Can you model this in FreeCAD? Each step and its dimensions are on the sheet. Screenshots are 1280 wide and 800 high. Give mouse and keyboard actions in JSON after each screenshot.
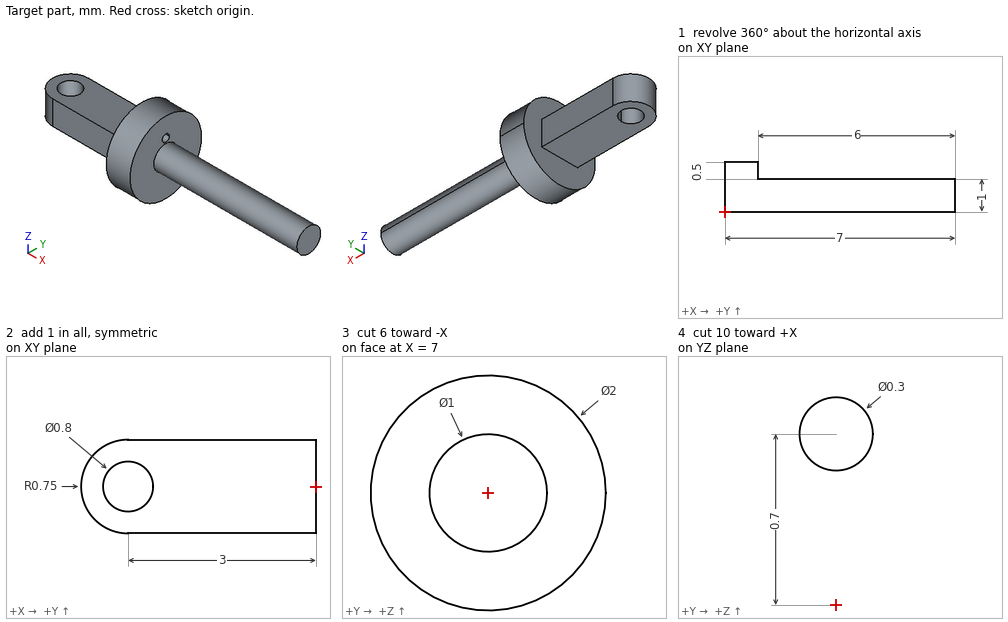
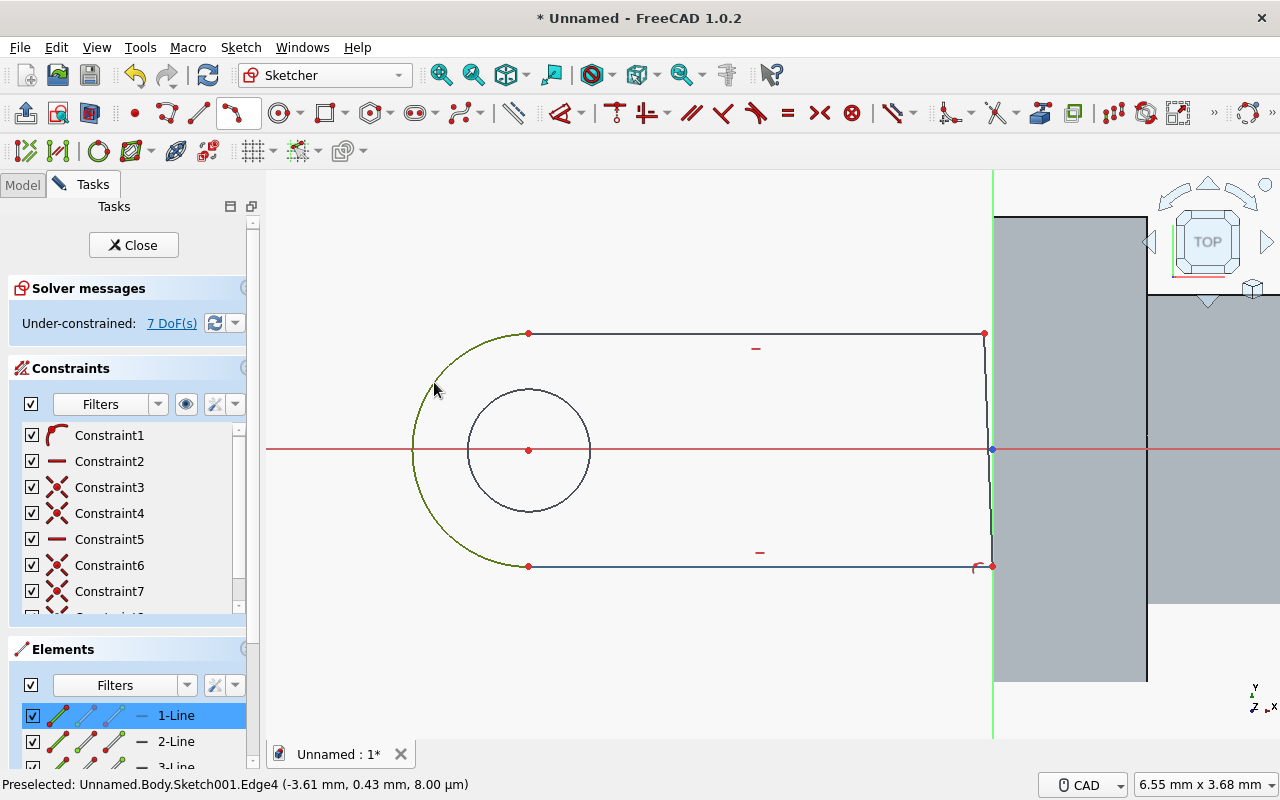
{"action": "left_click", "coordinate": [756, 114]}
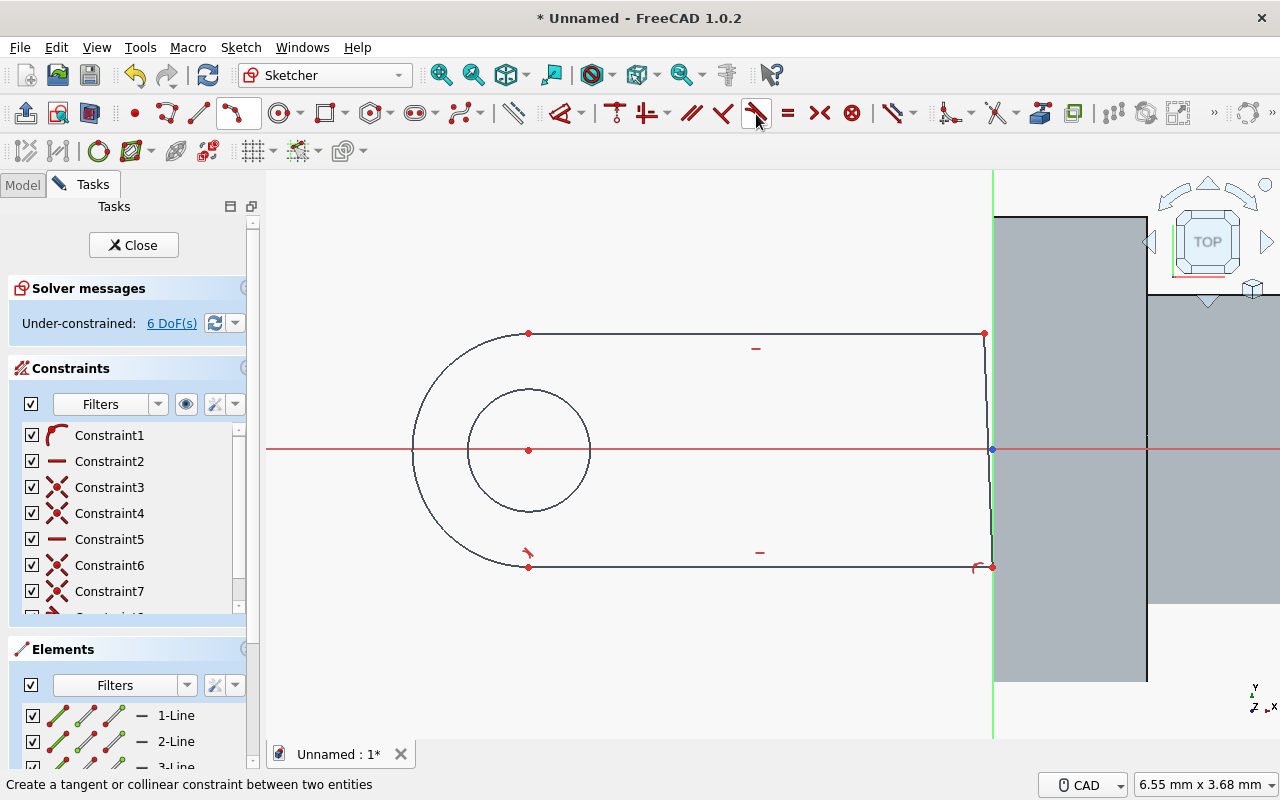
{"action": "left_click", "coordinate": [847, 334]}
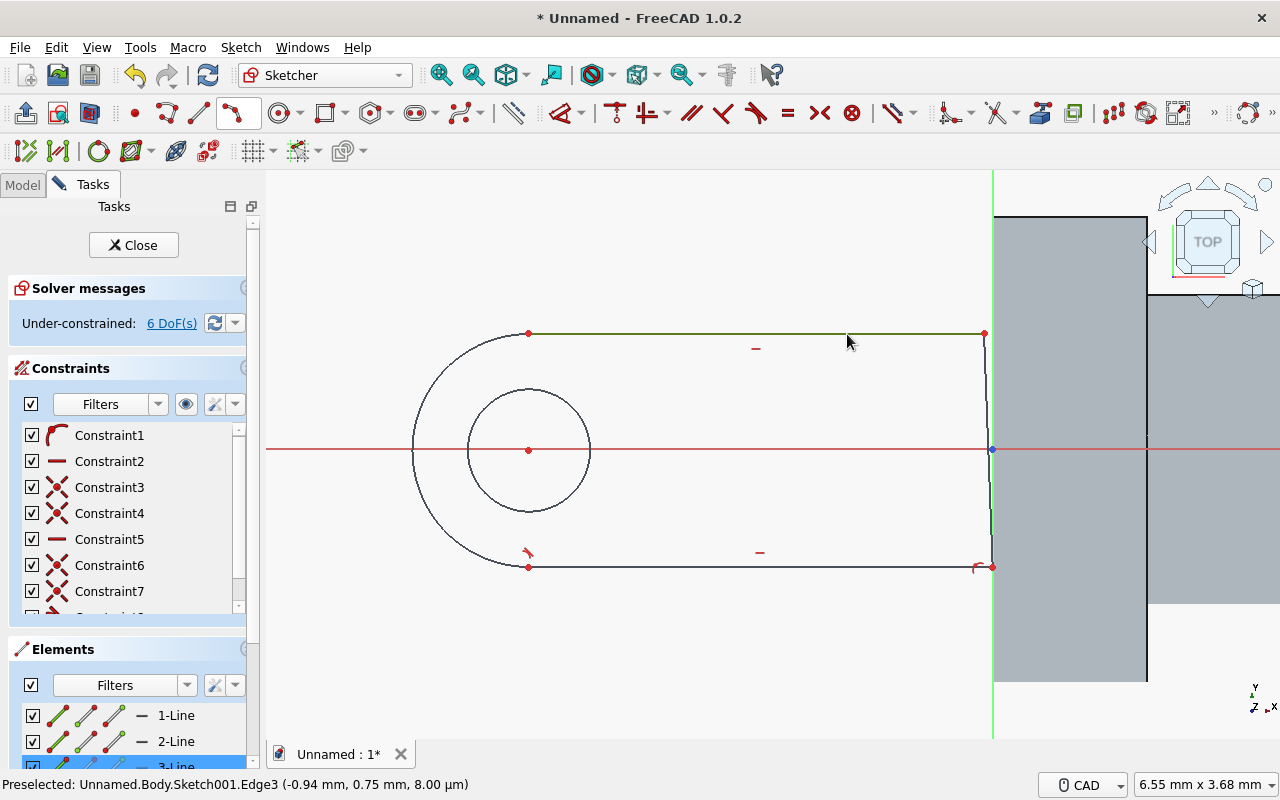
{"action": "left_click", "coordinate": [434, 383]}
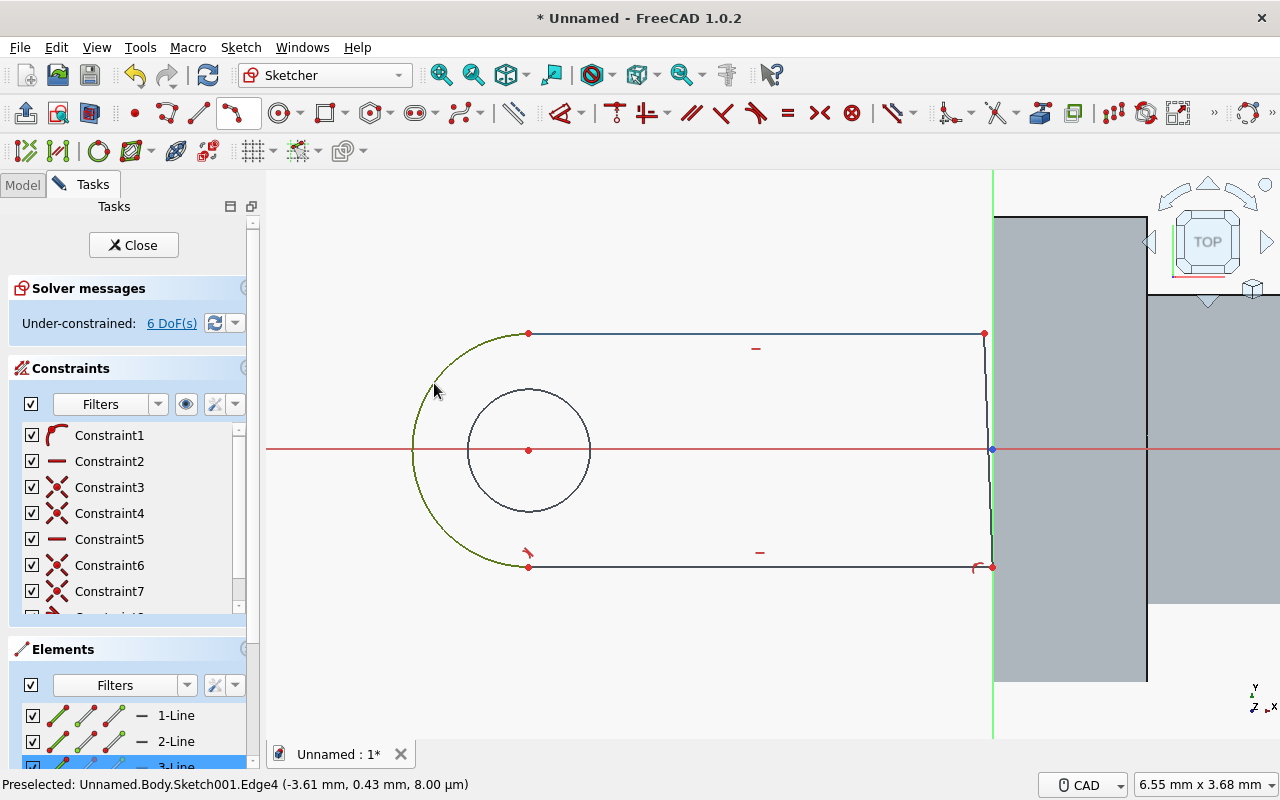
{"action": "left_click", "coordinate": [756, 114]}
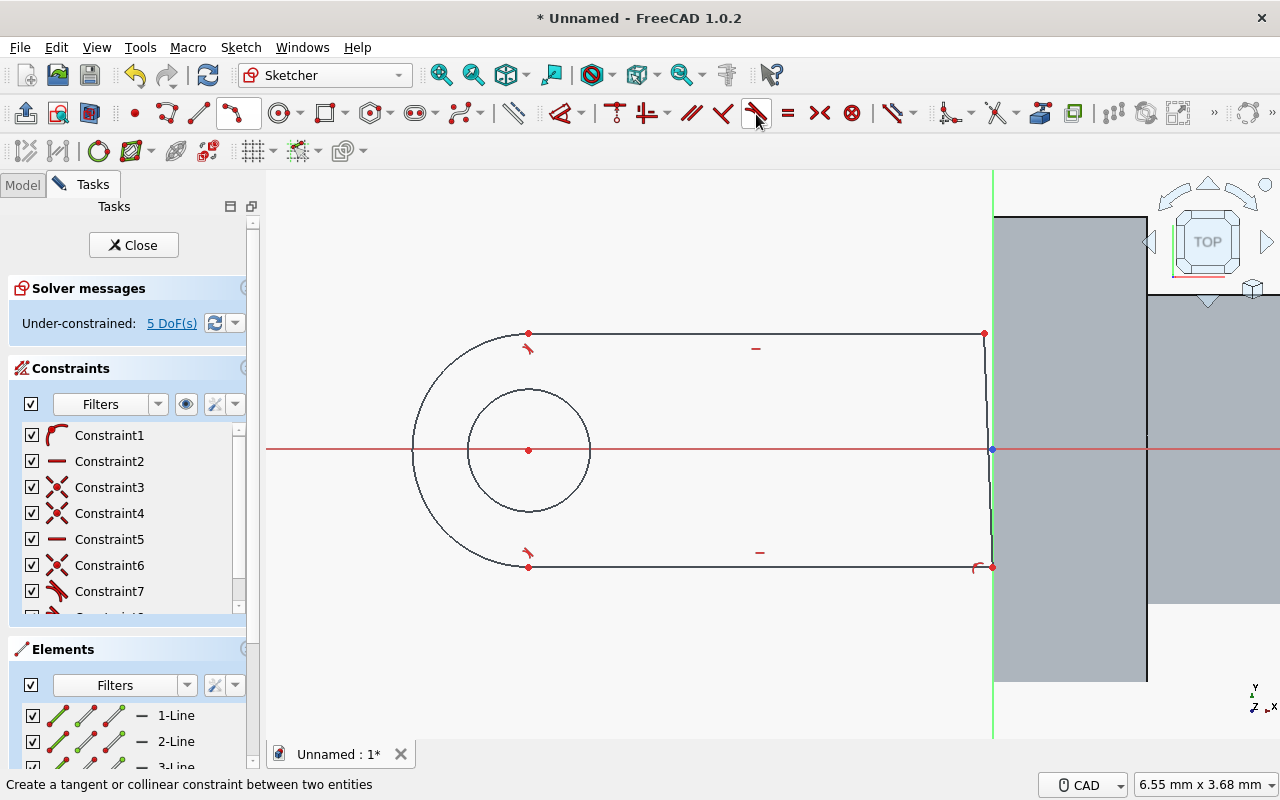
{"action": "left_click", "coordinate": [990, 497]}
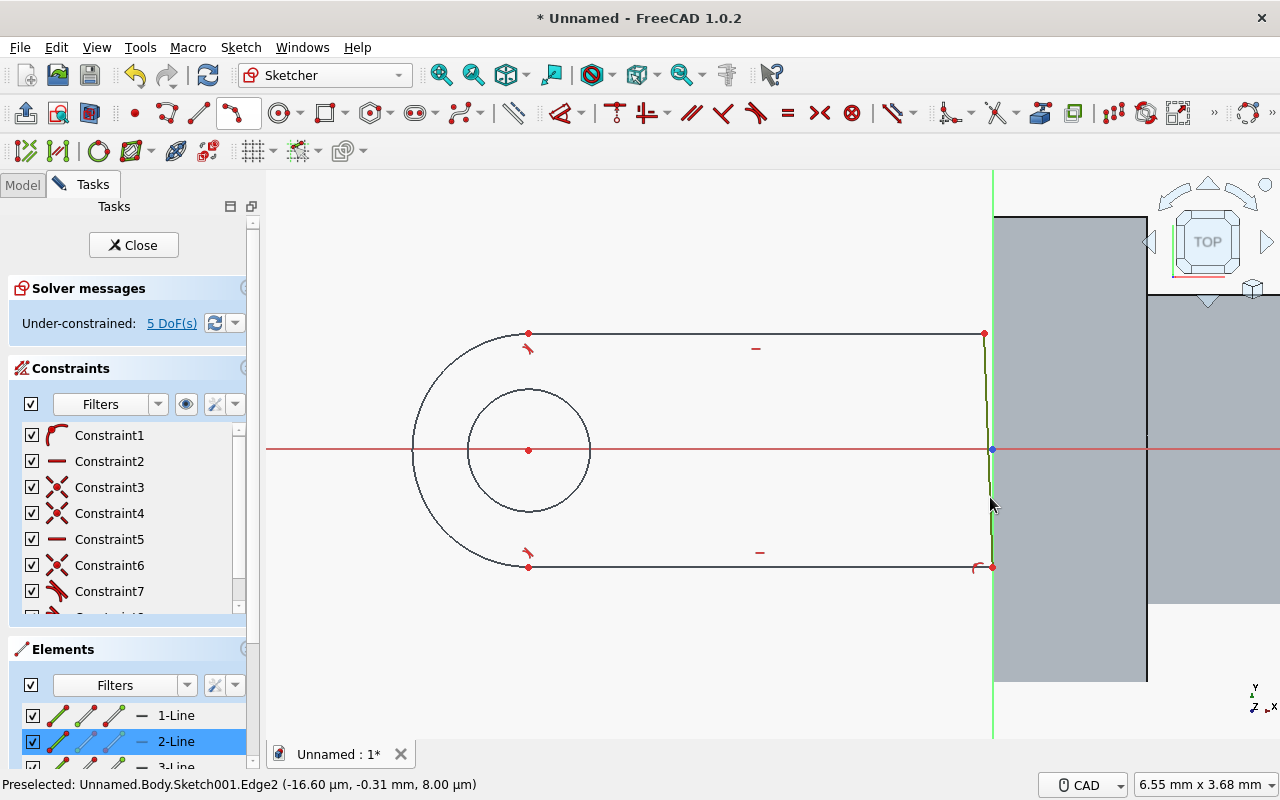
{"action": "left_click", "coordinate": [670, 114]}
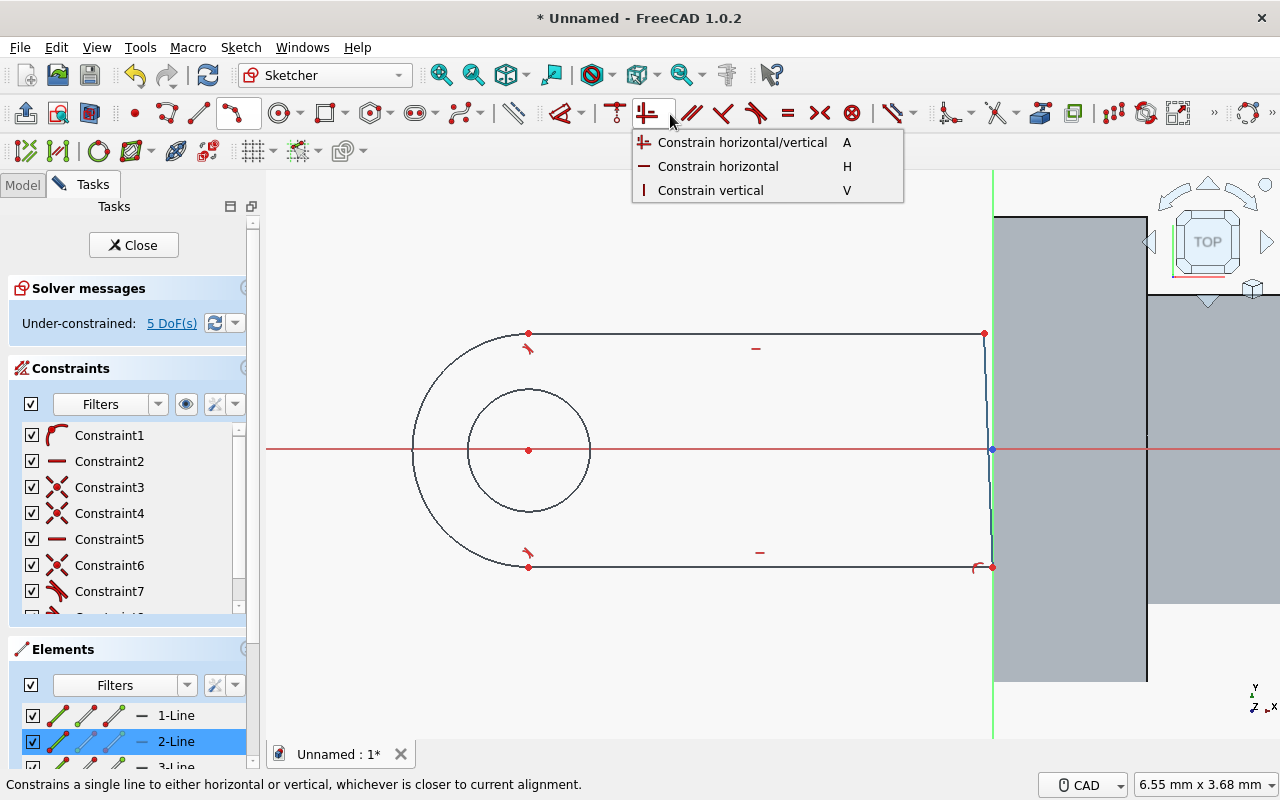
{"action": "left_click", "coordinate": [768, 190]}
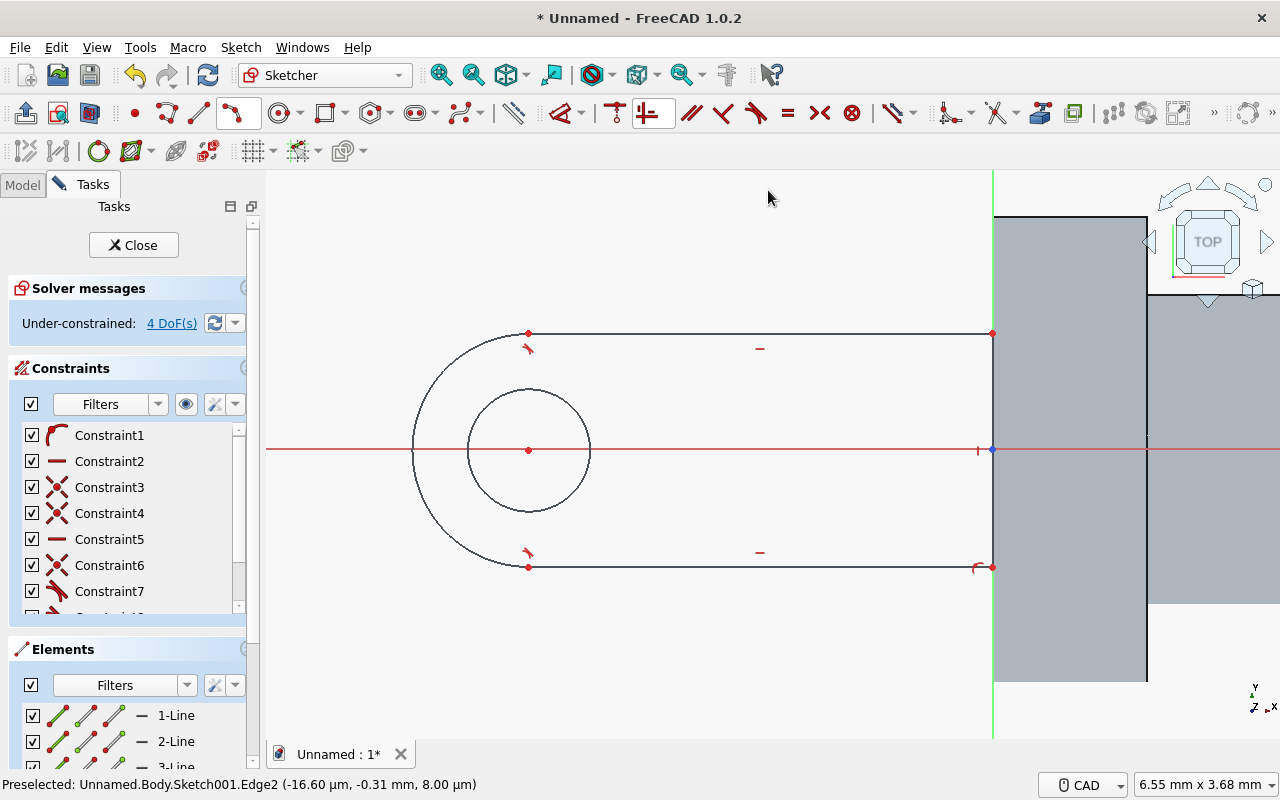
{"action": "left_click", "coordinate": [529, 451]}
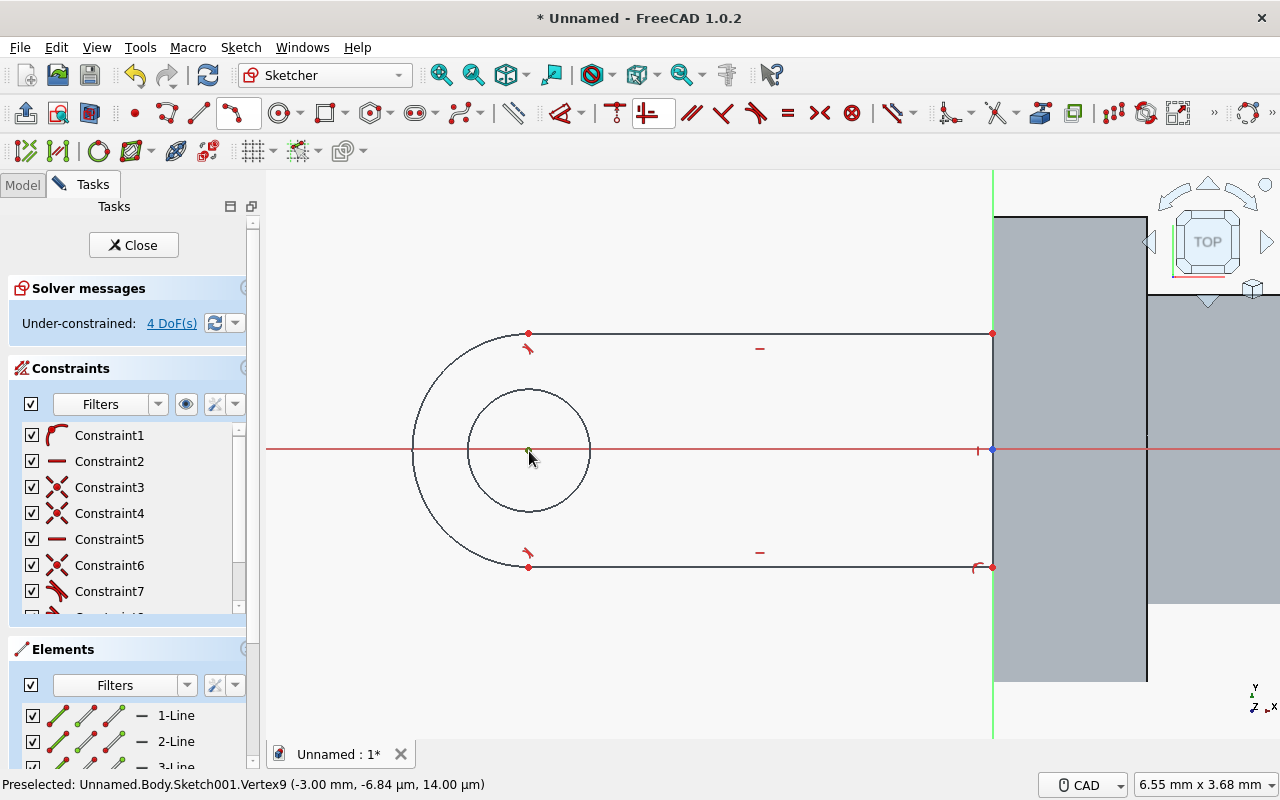
{"action": "left_click", "coordinate": [353, 449]}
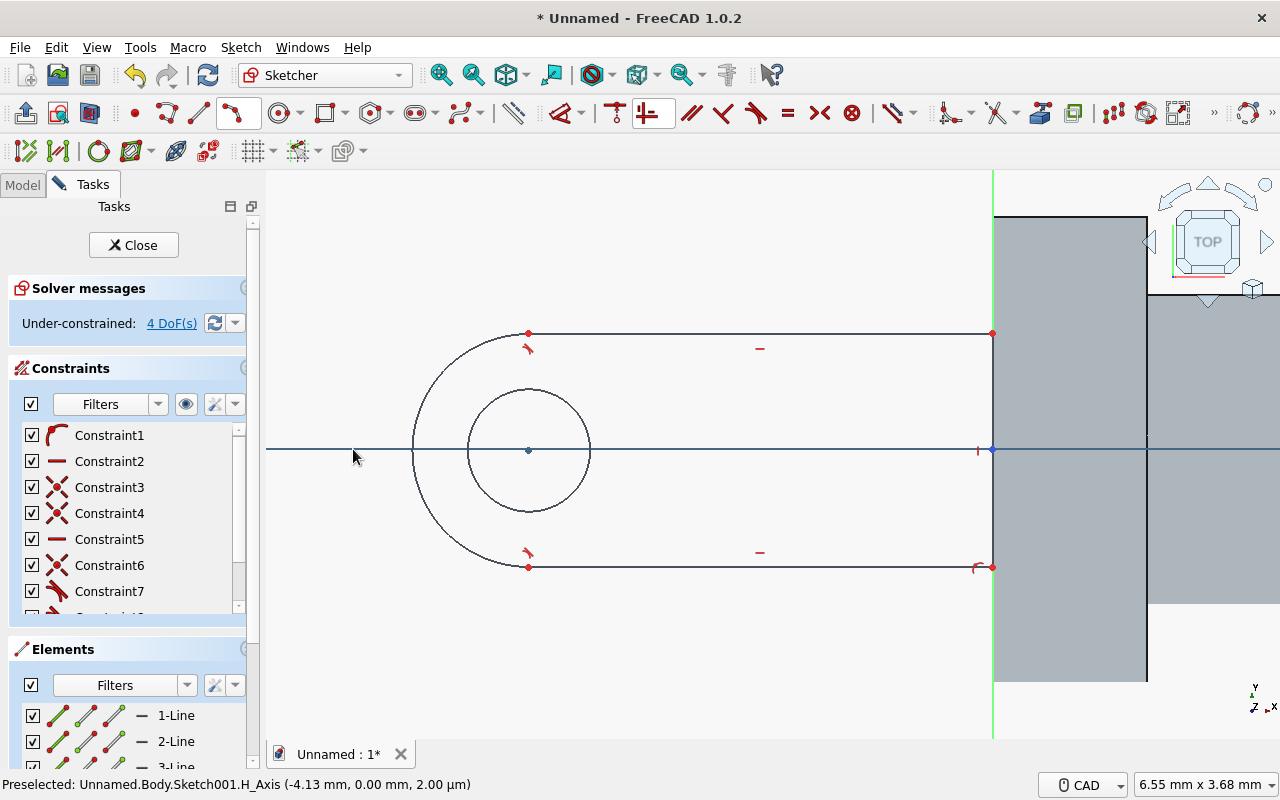
{"action": "left_click", "coordinate": [616, 114]}